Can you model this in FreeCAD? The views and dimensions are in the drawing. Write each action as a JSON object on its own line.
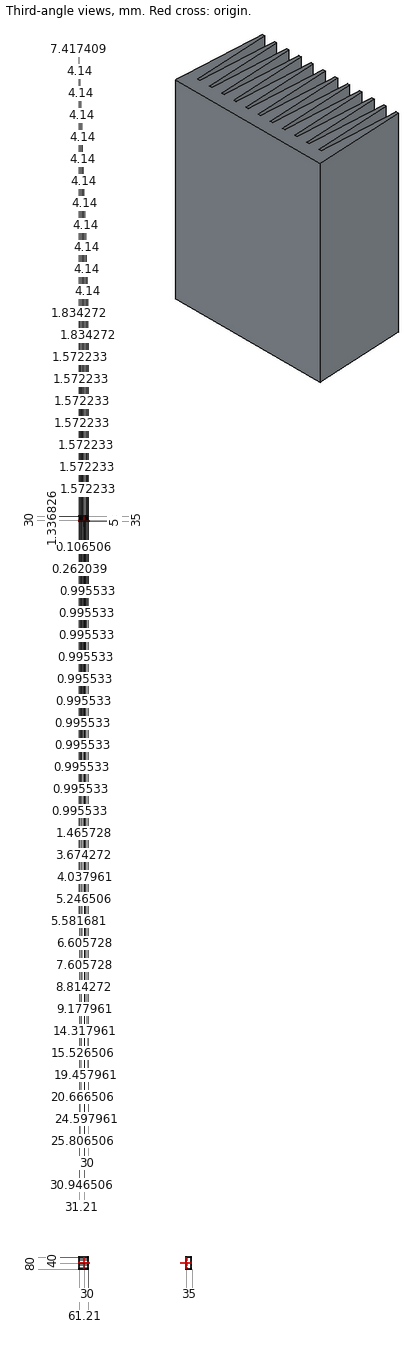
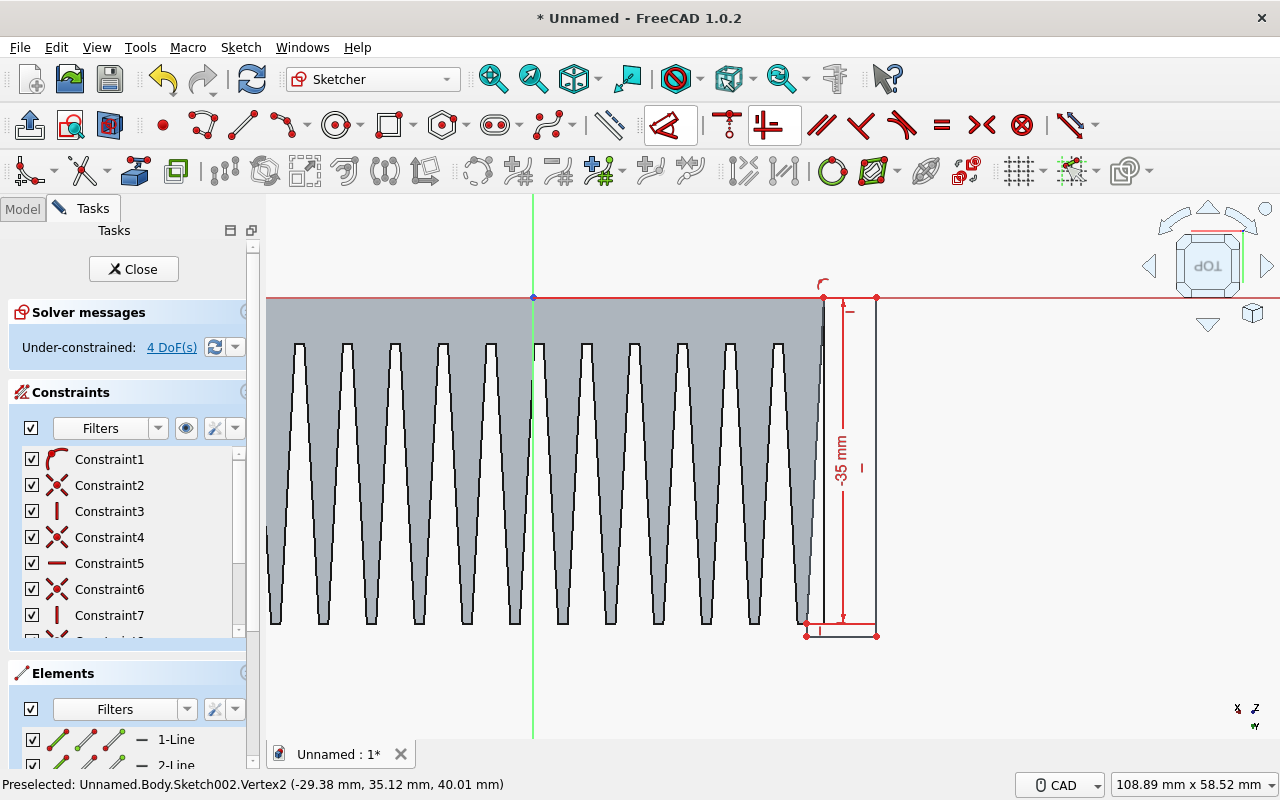
{"action": "left_click", "coordinate": [824, 298]}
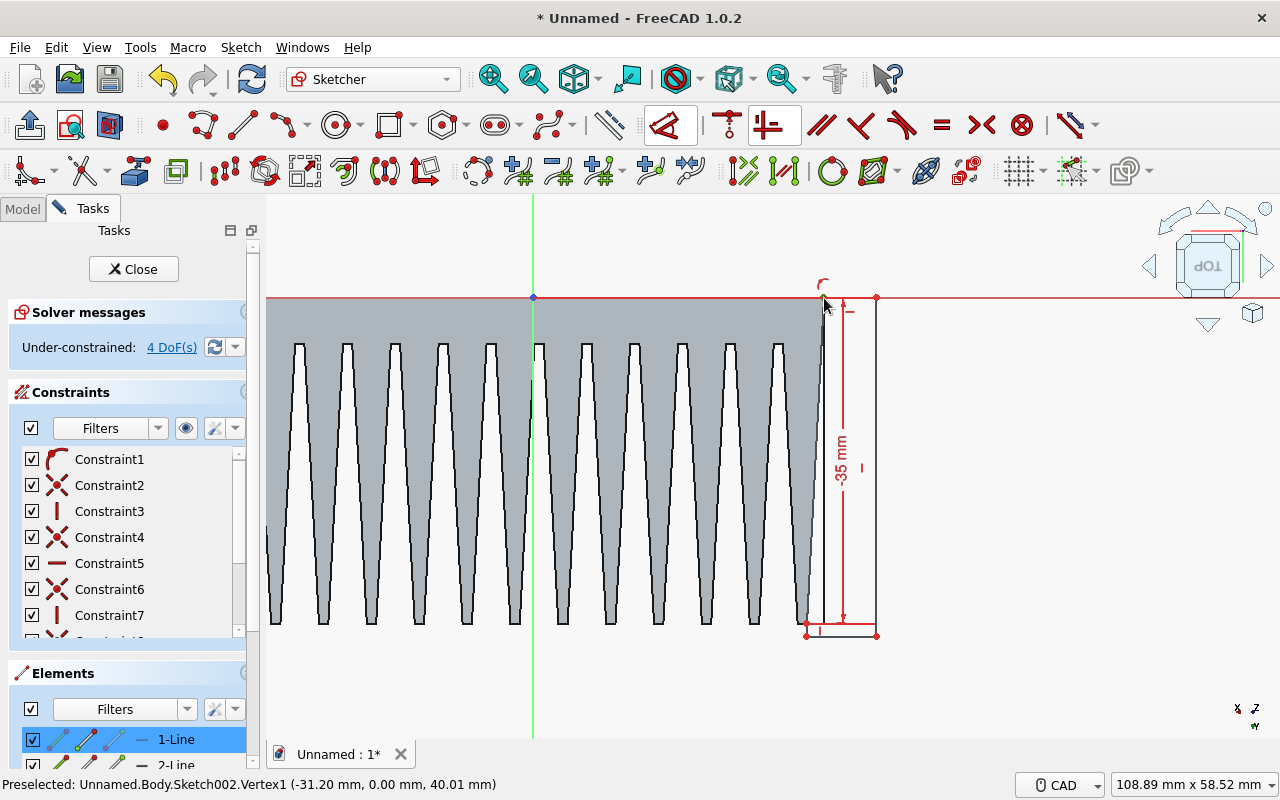
{"action": "key", "text": "l"}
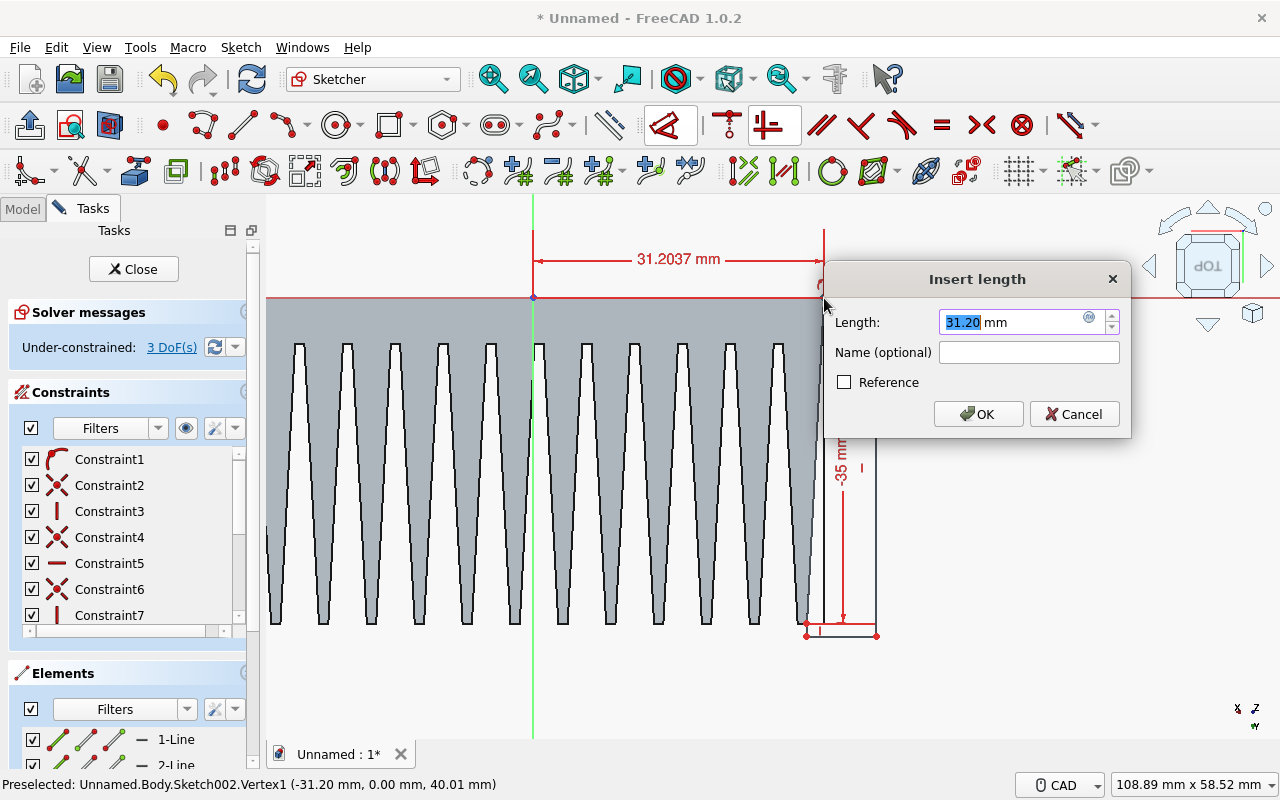
{"action": "type", "text": "31.21"}
{"action": "key", "text": "Return"}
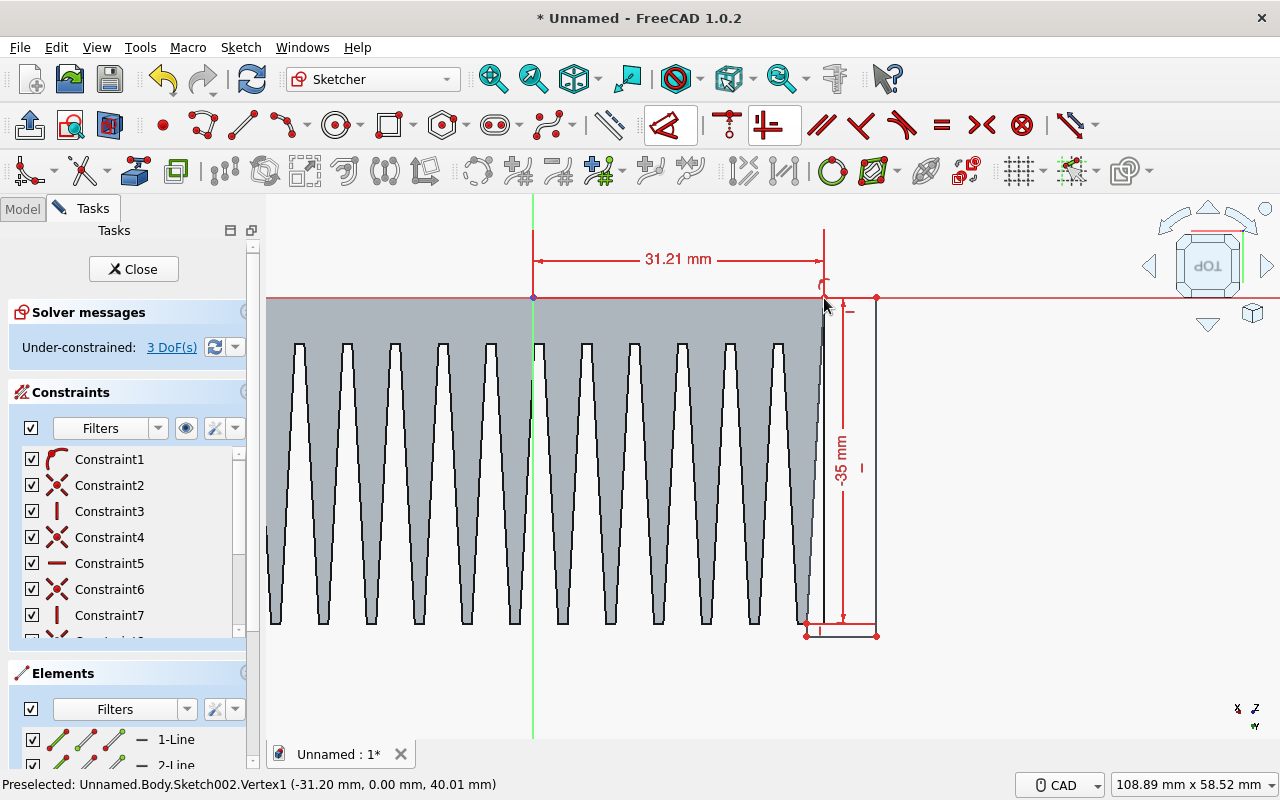
{"action": "scroll", "coordinate": [807, 630], "scroll_direction": "up", "scroll_amount": 6}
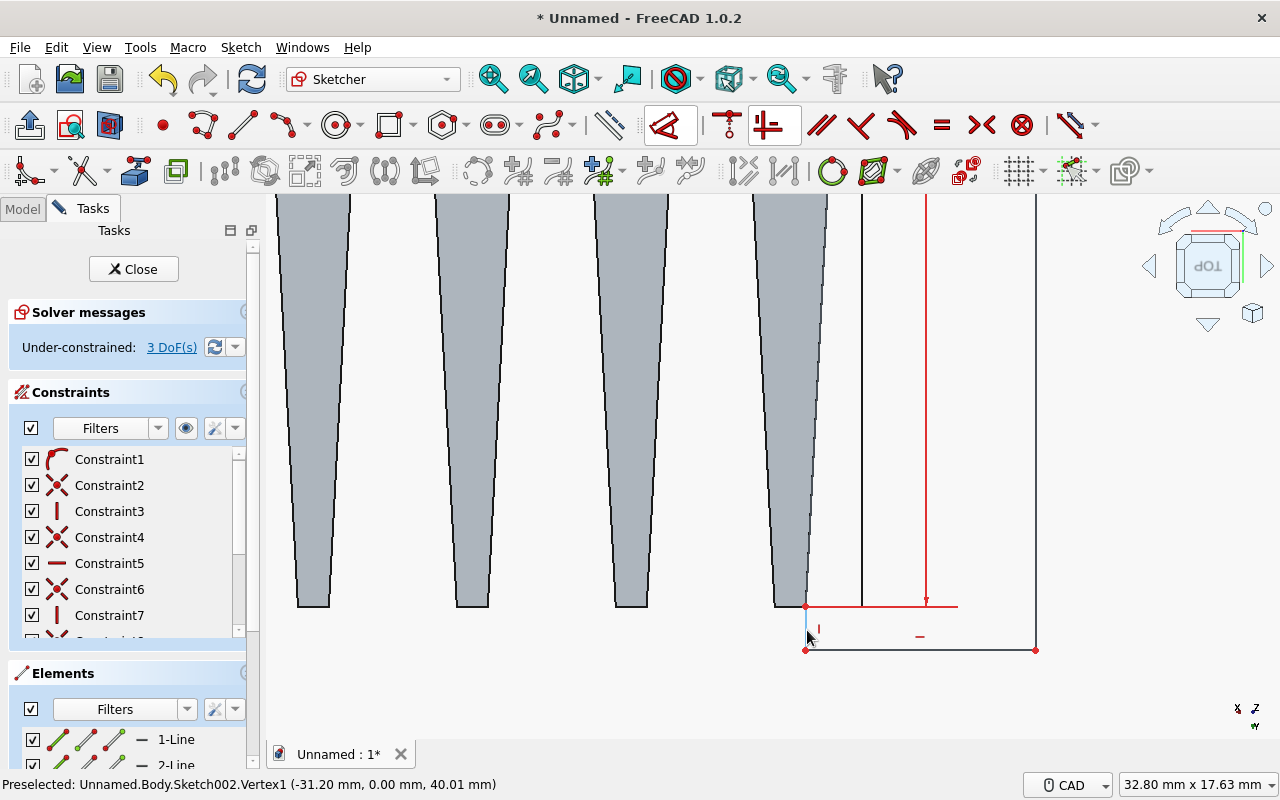
{"action": "left_click", "coordinate": [806, 628]}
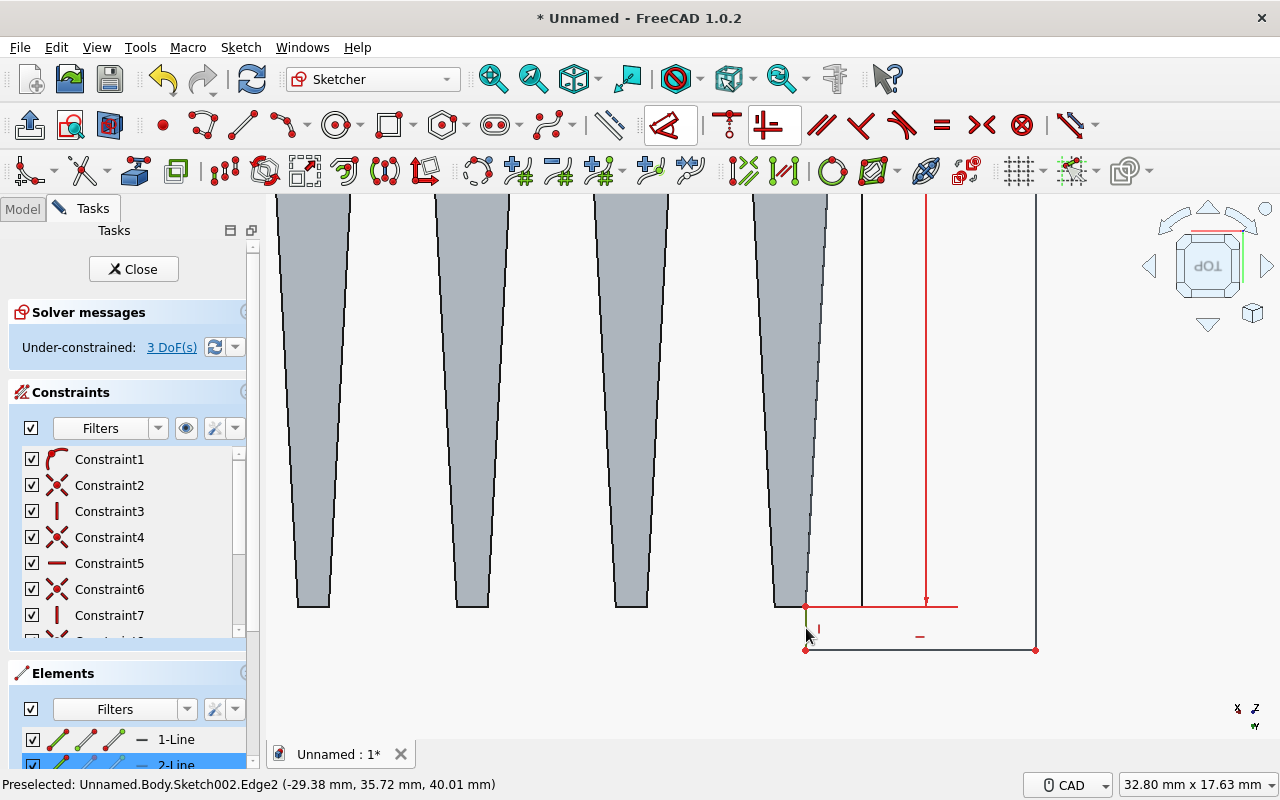
{"action": "left_click", "coordinate": [692, 126]}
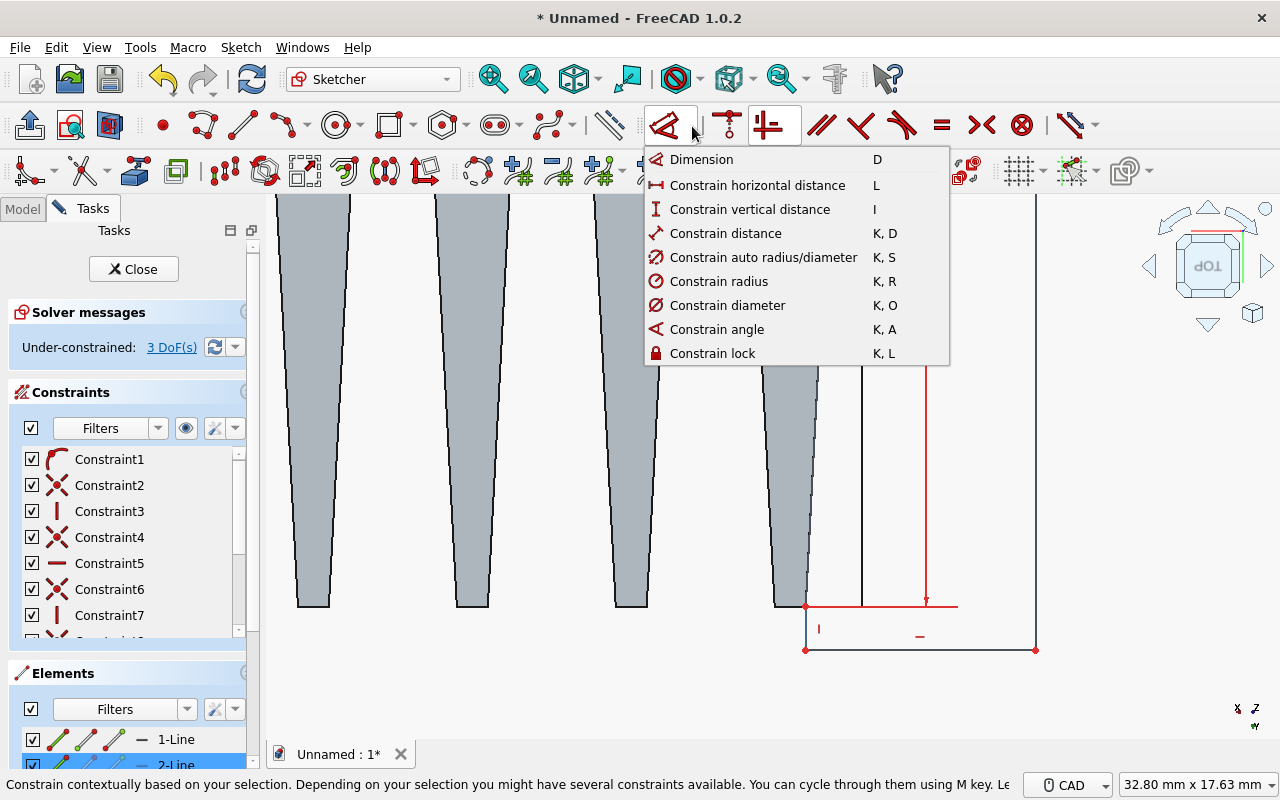
{"action": "left_click", "coordinate": [797, 209]}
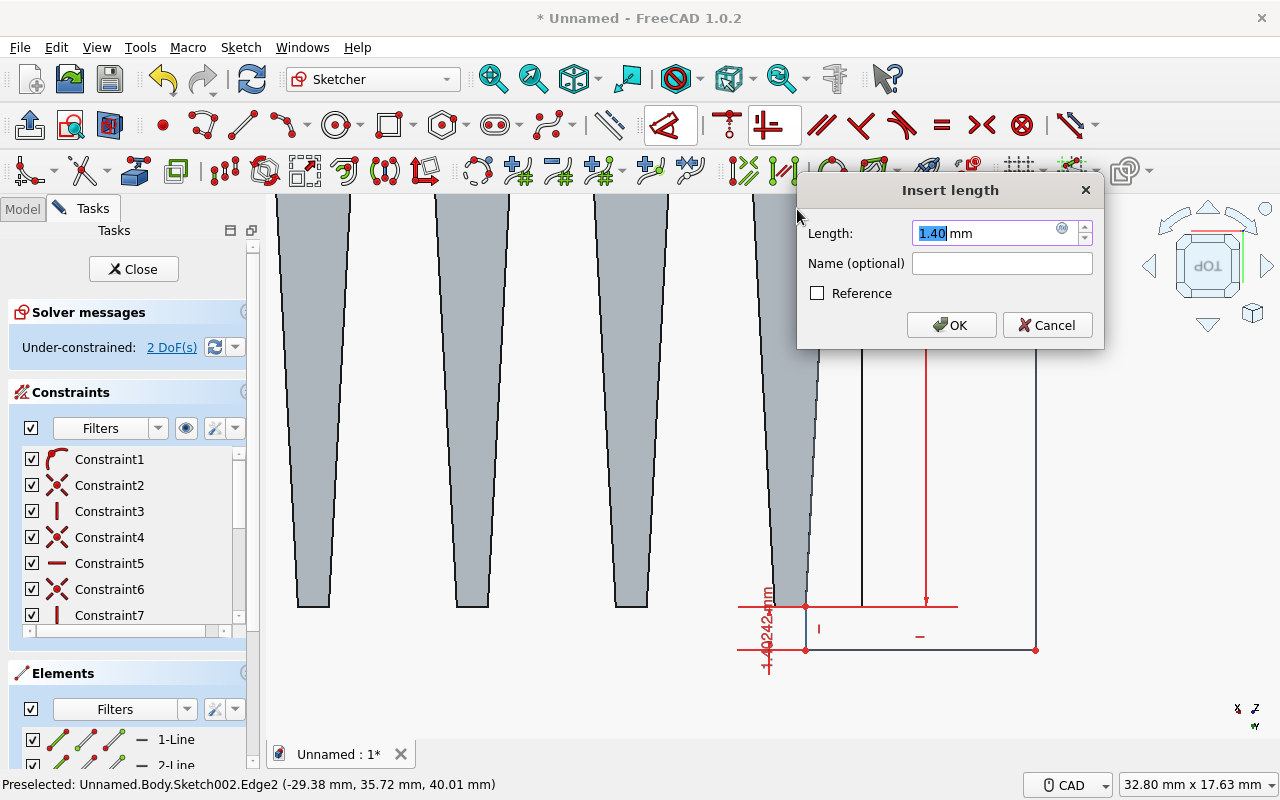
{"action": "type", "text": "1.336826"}
{"action": "key", "text": "Return"}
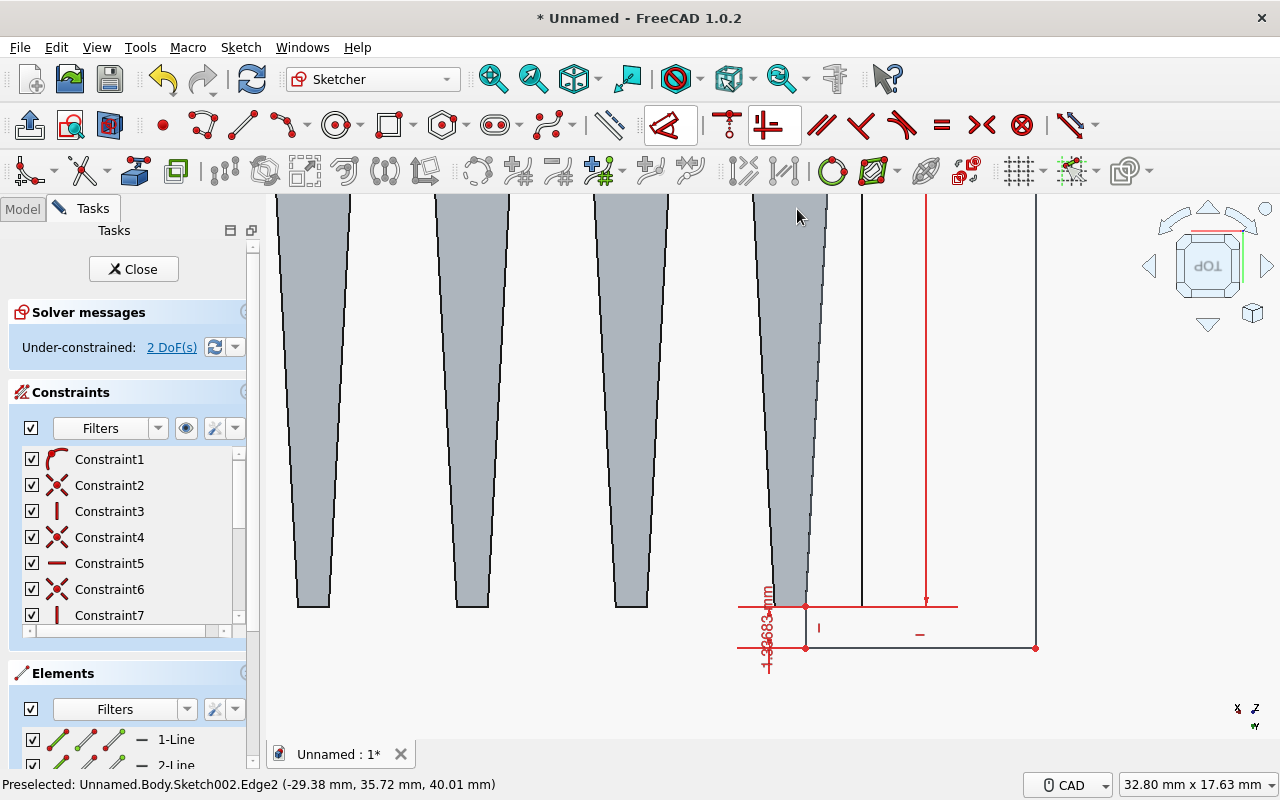
{"action": "left_click", "coordinate": [875, 648]}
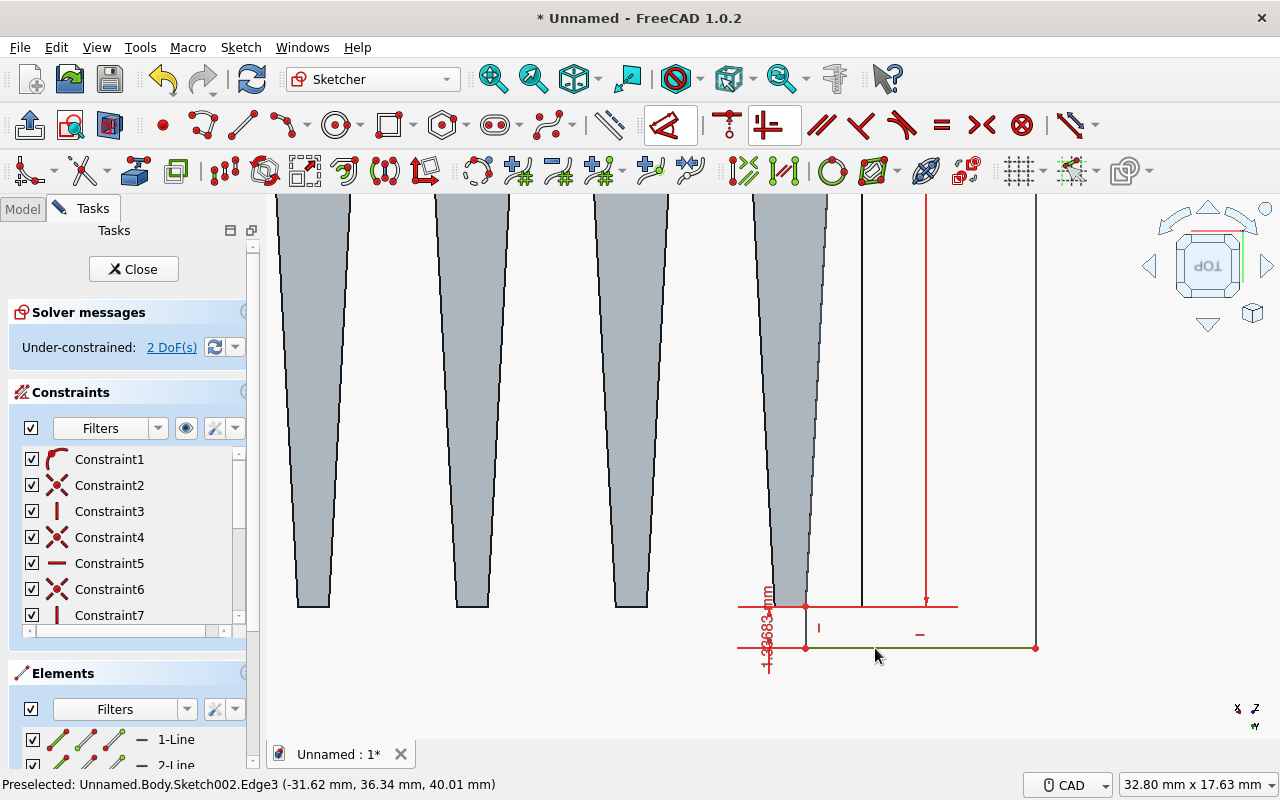
{"action": "key", "text": "l"}